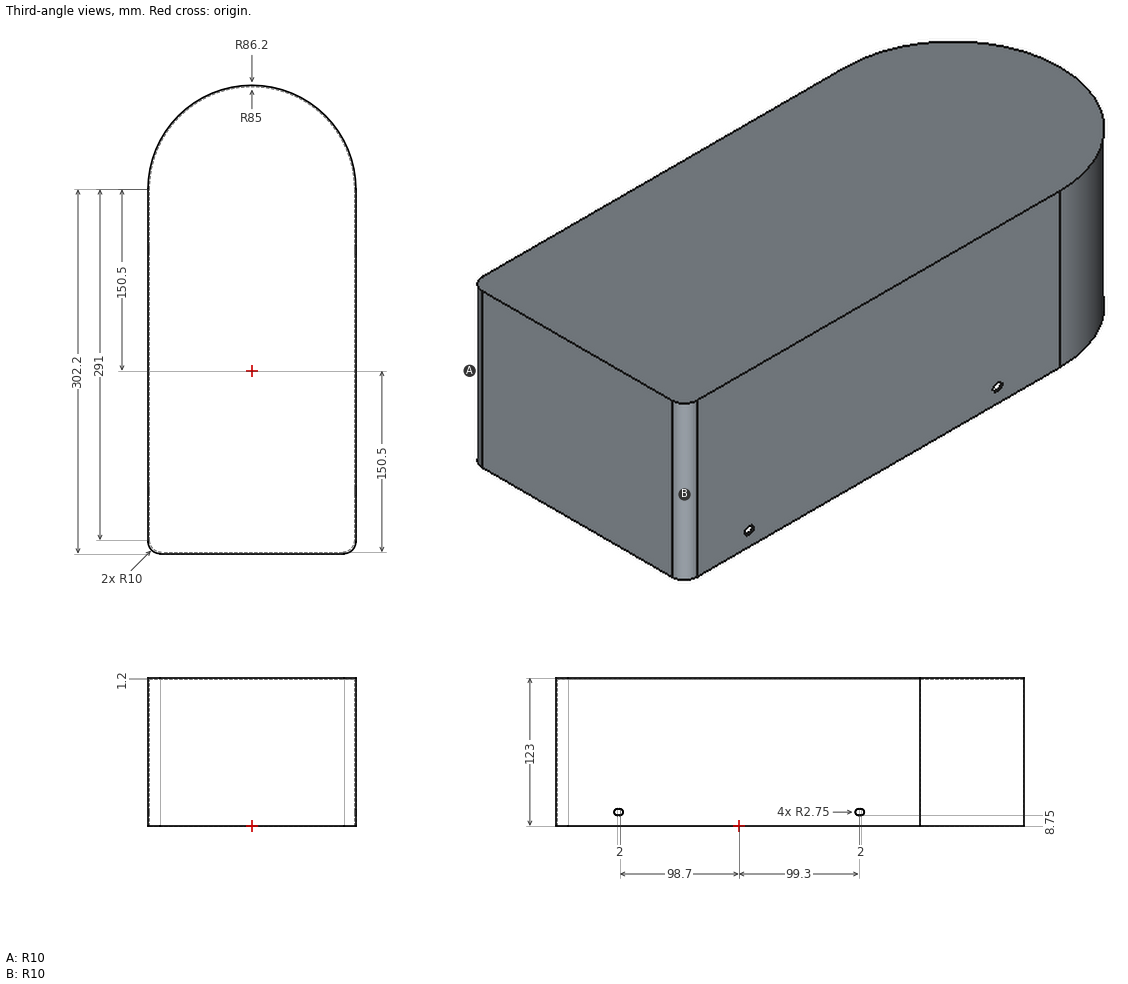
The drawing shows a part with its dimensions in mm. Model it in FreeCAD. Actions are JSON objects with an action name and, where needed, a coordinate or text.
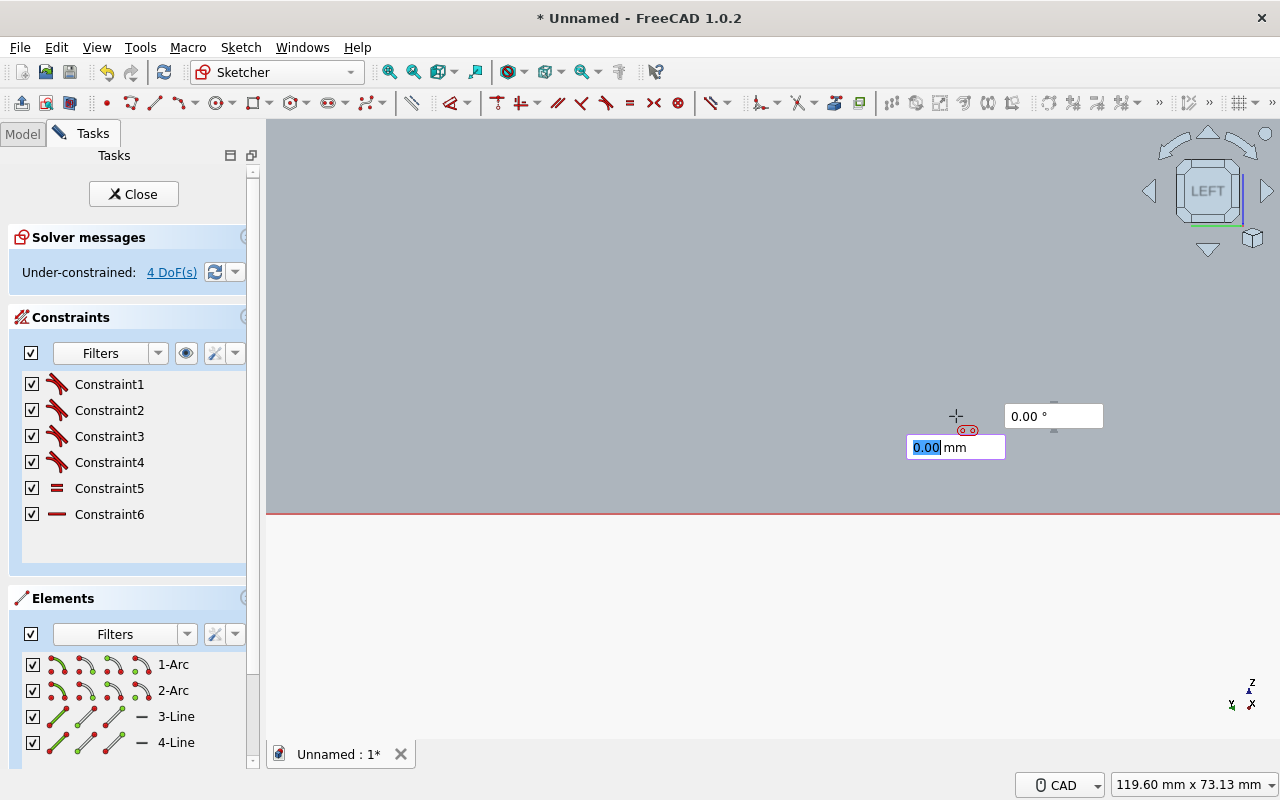
{"action": "left_click", "coordinate": [973, 416]}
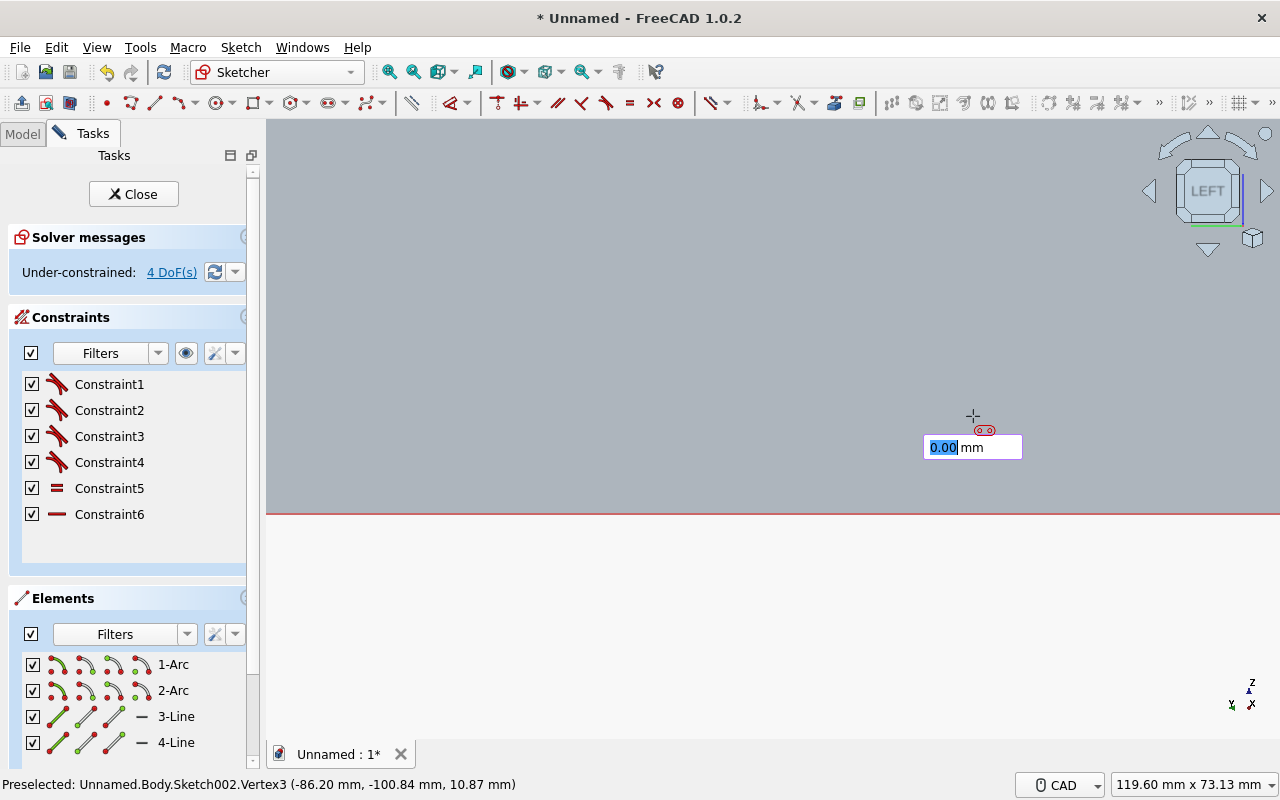
{"action": "left_click", "coordinate": [964, 440]}
{"action": "key", "text": "Escape"}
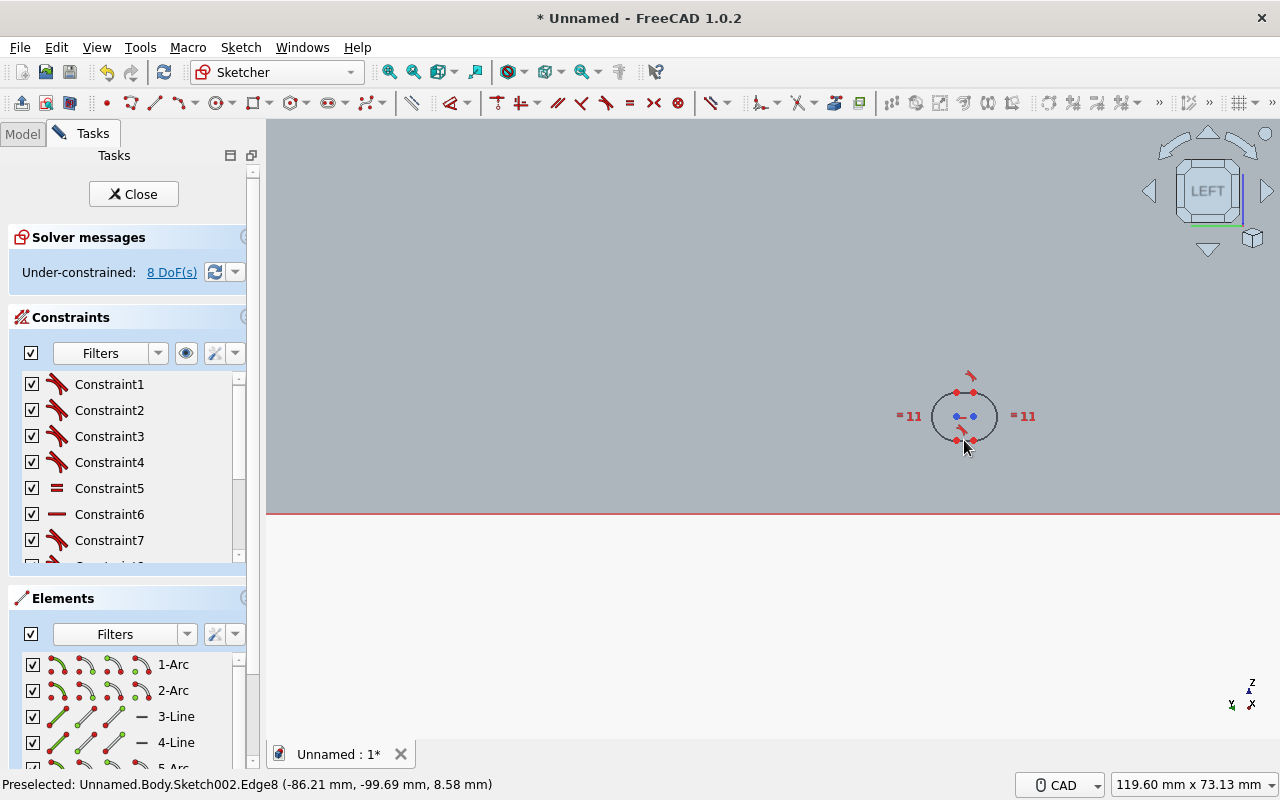
{"action": "scroll", "coordinate": [958, 419], "scroll_direction": "down", "scroll_amount": 6}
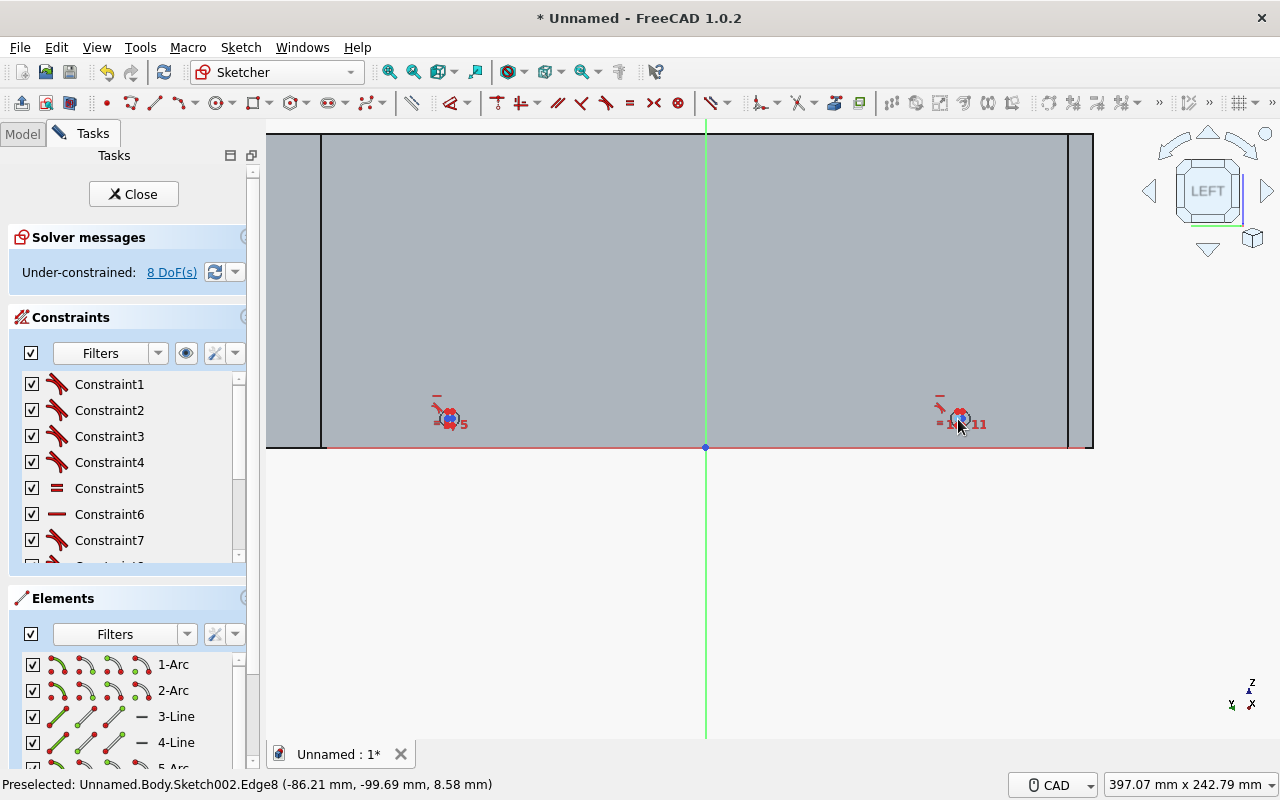
{"action": "scroll", "coordinate": [441, 414], "scroll_direction": "up", "scroll_amount": 4}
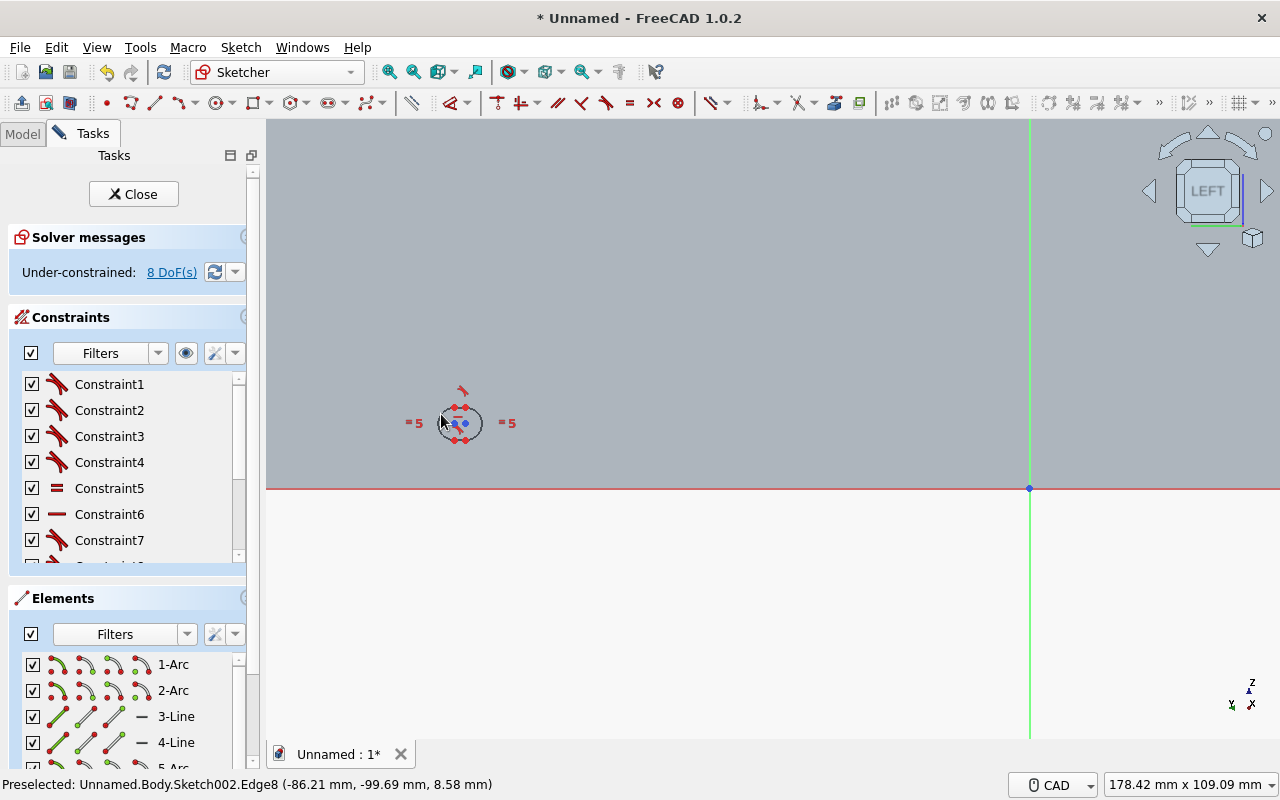
{"action": "left_click", "coordinate": [441, 415]}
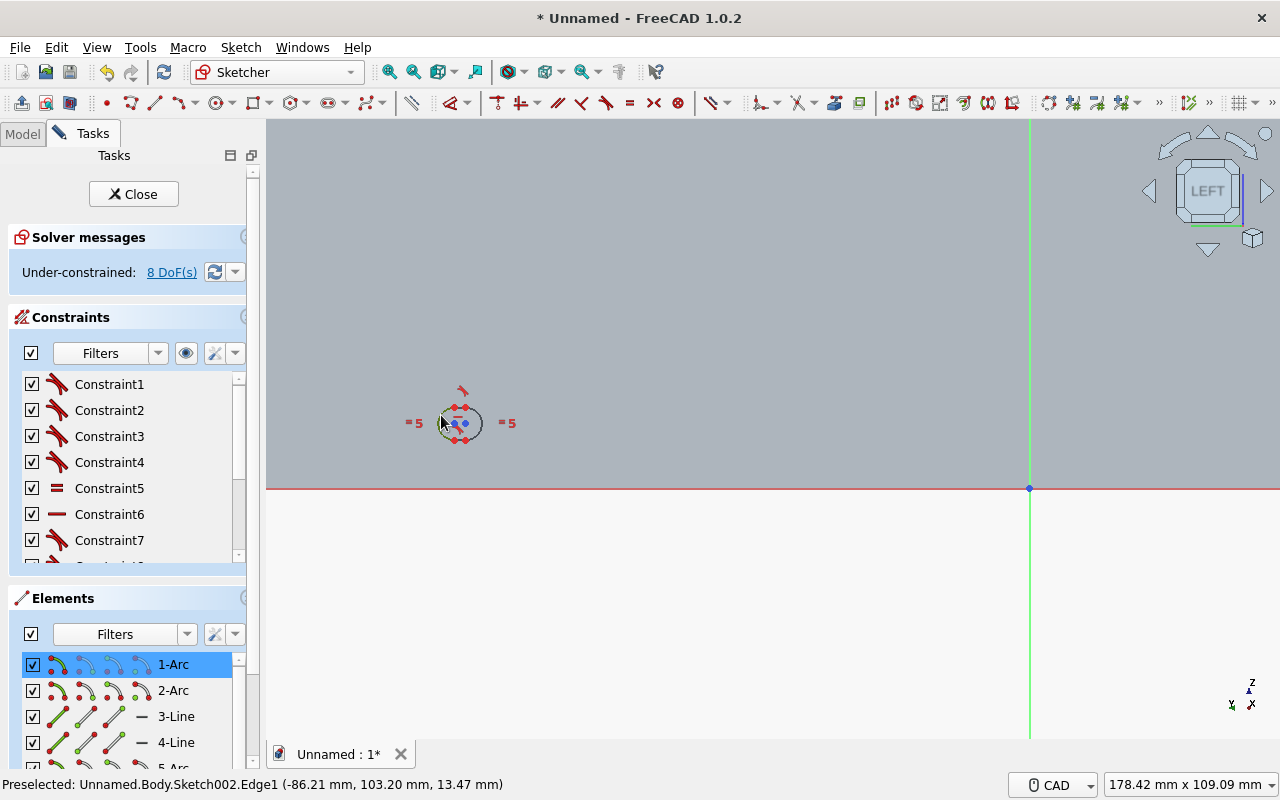
{"action": "scroll", "coordinate": [440, 413], "scroll_direction": "down", "scroll_amount": 4}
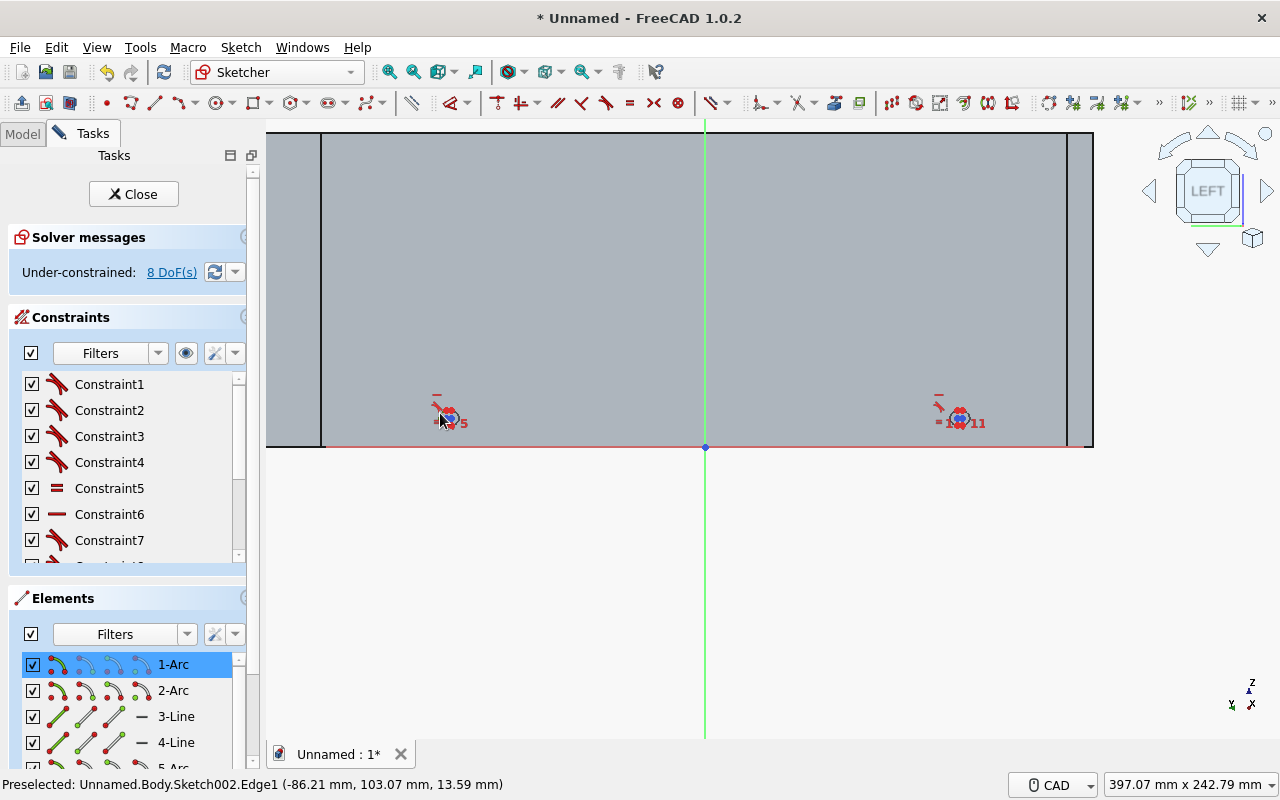
{"action": "scroll", "coordinate": [951, 414], "scroll_direction": "up", "scroll_amount": 4}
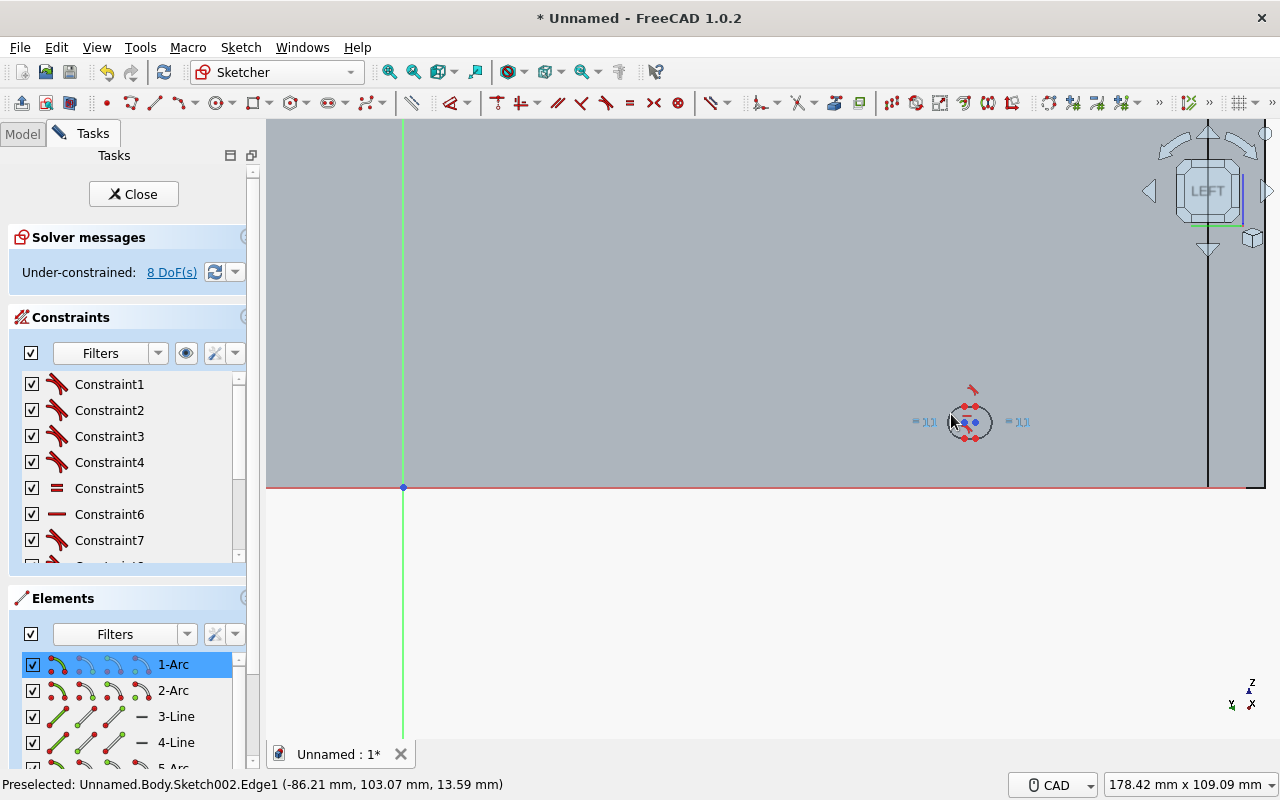
{"action": "left_click", "coordinate": [951, 413]}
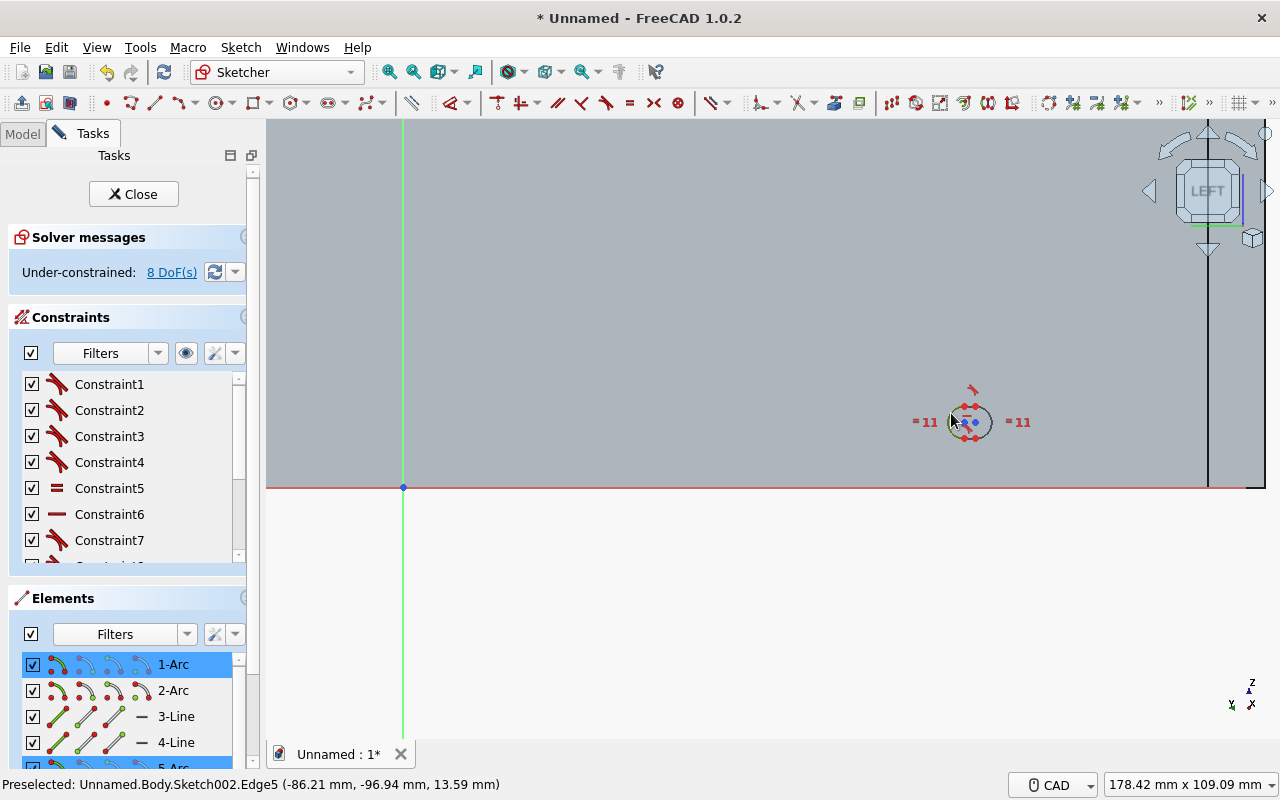
{"action": "left_click", "coordinate": [630, 104]}